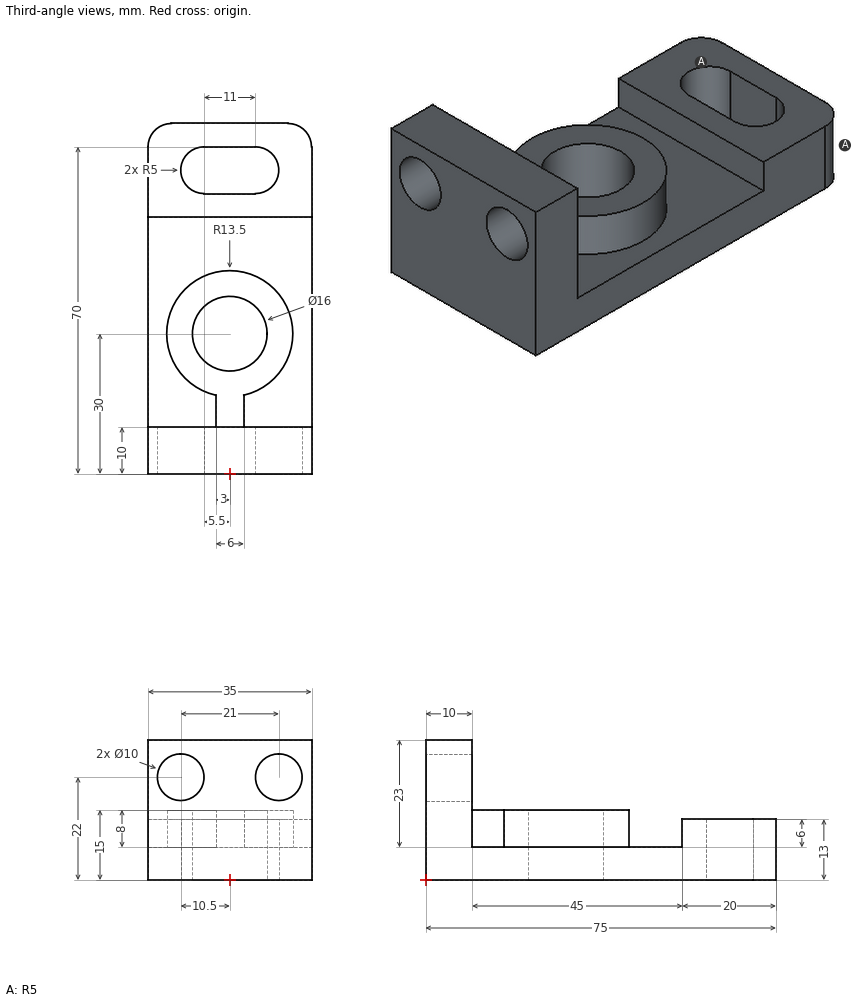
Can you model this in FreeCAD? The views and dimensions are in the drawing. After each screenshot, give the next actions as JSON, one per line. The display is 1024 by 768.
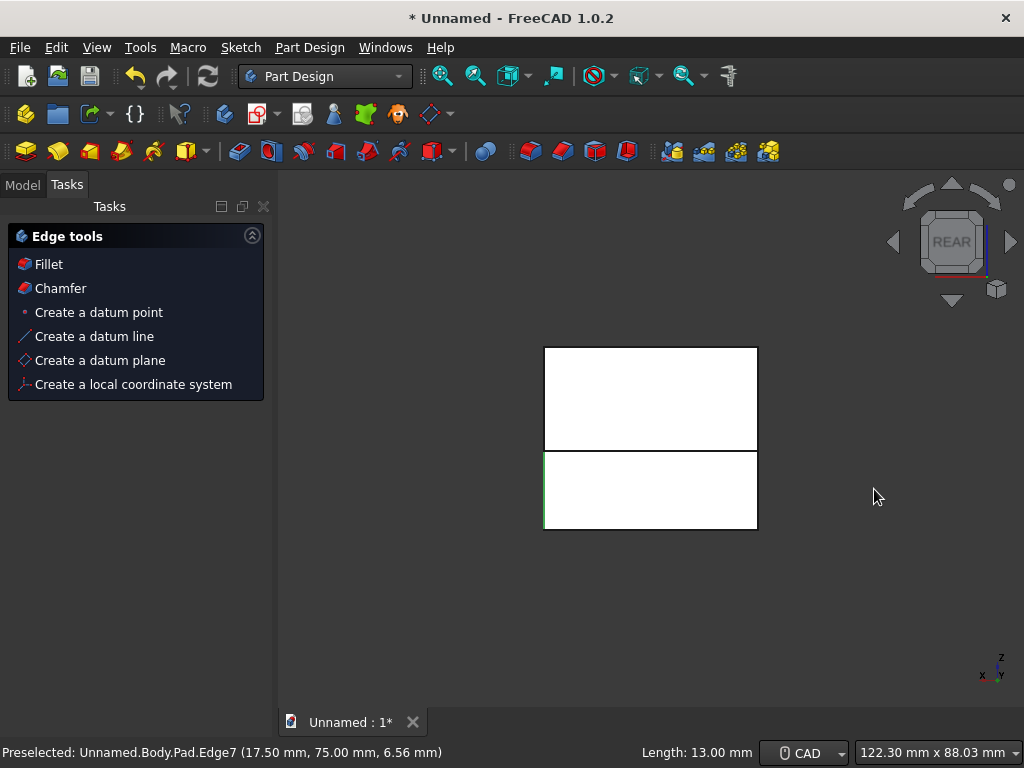
{"action": "key", "text": "v f"}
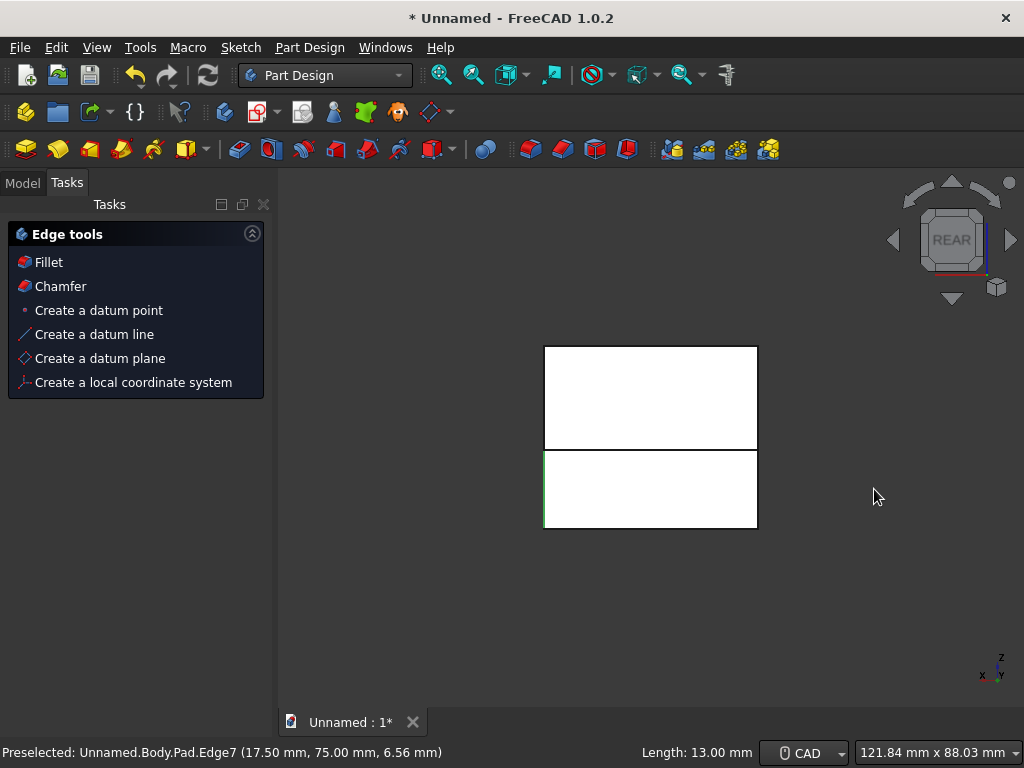
{"action": "left_click", "coordinate": [758, 489], "text": "ctrl"}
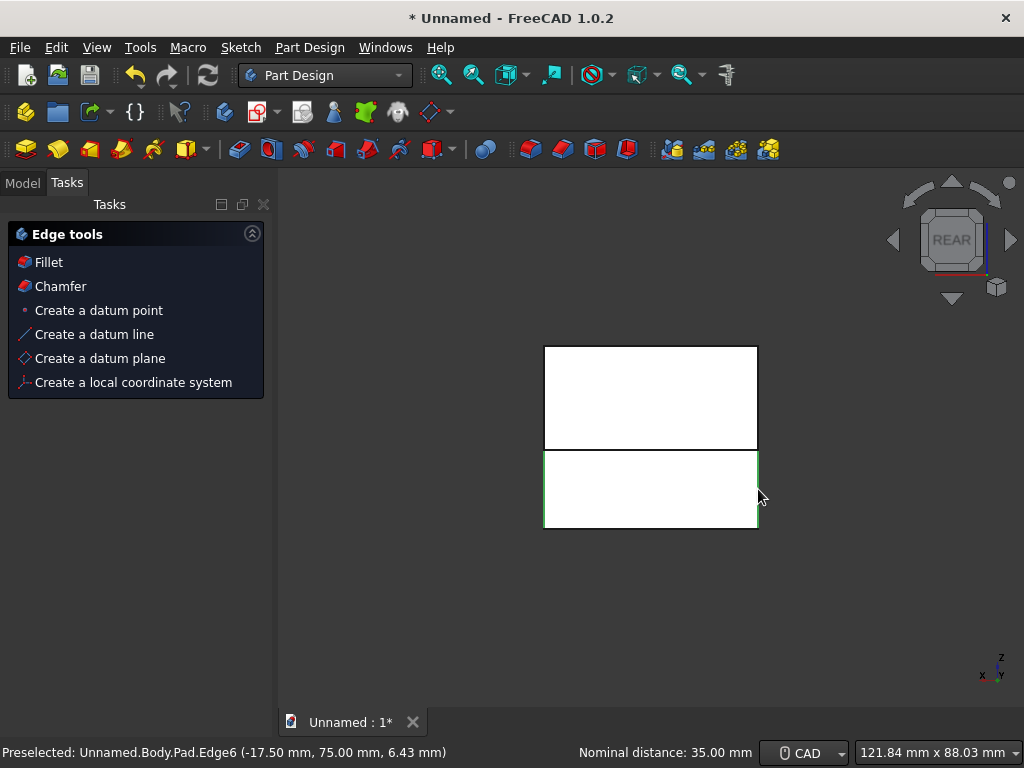
{"action": "left_click", "coordinate": [532, 150]}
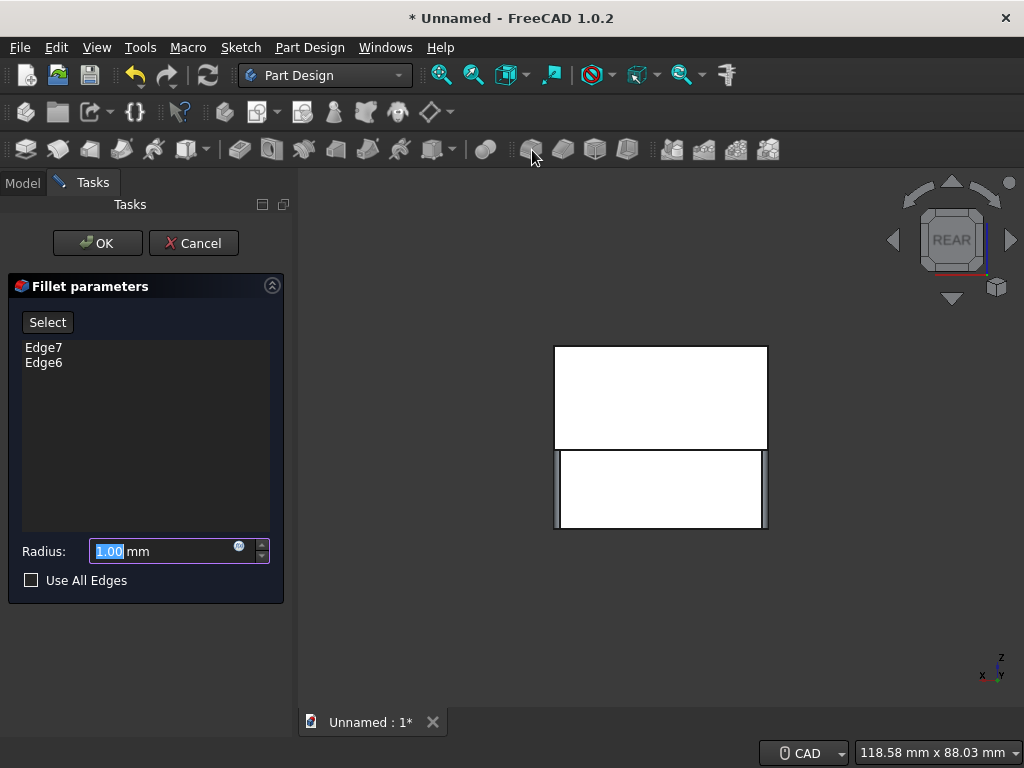
{"action": "type", "text": "5"}
{"action": "key", "text": "Tab"}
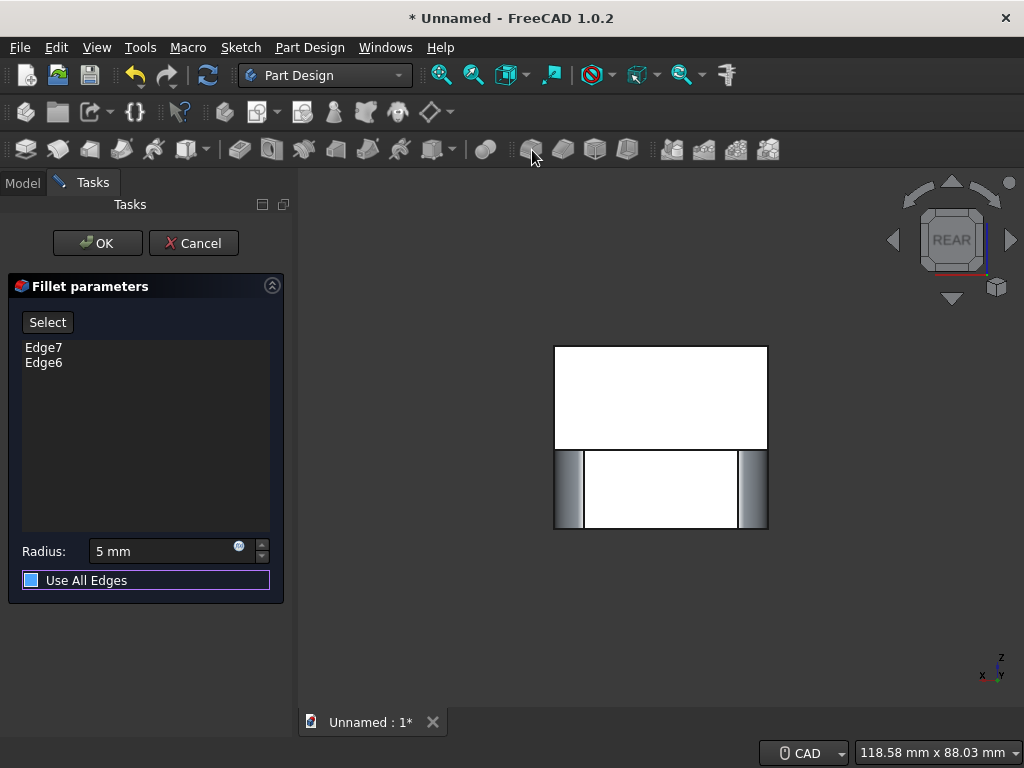
{"action": "left_click", "coordinate": [98, 243]}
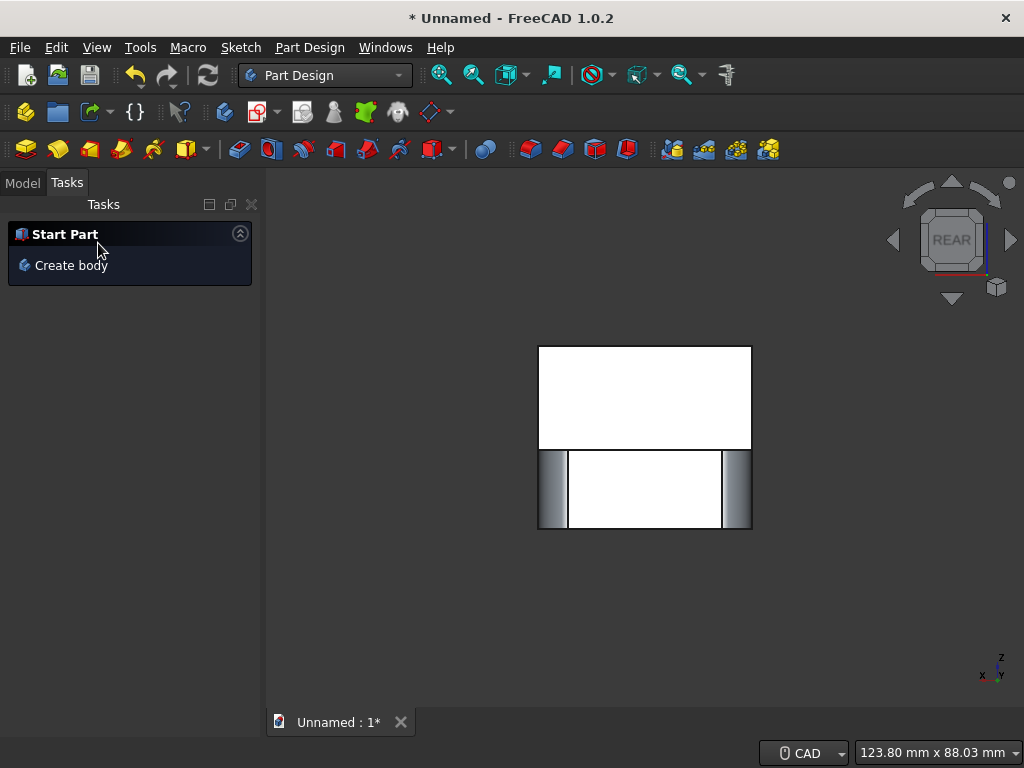
{"action": "key", "text": "v f"}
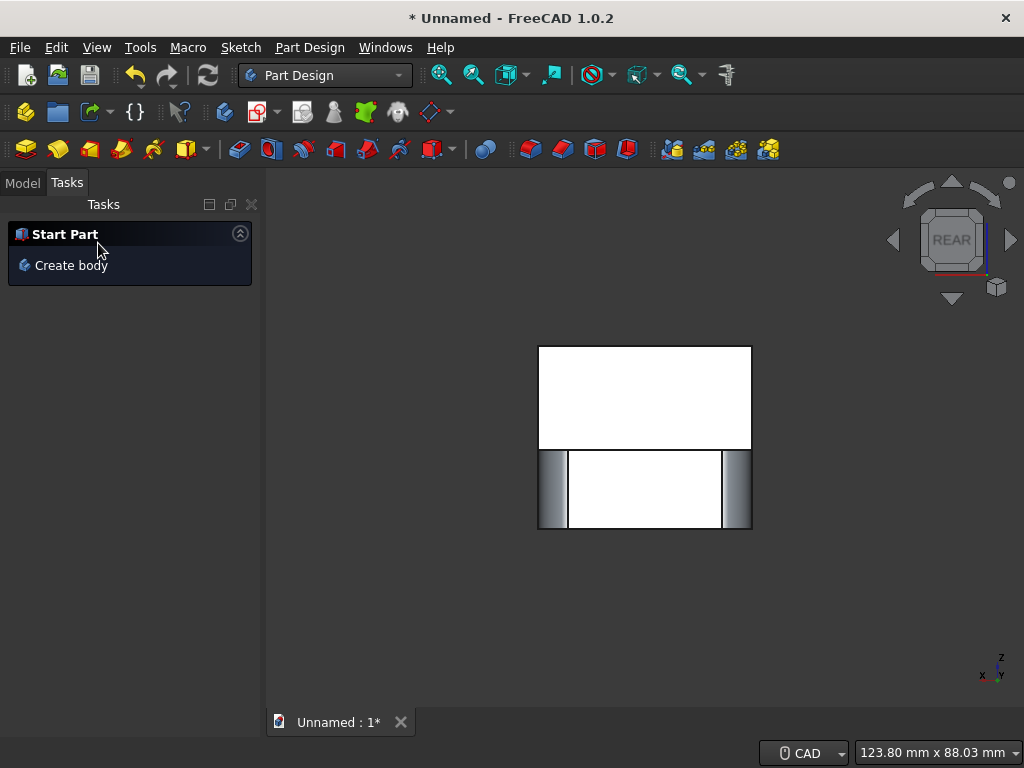
{"action": "key", "text": "0"}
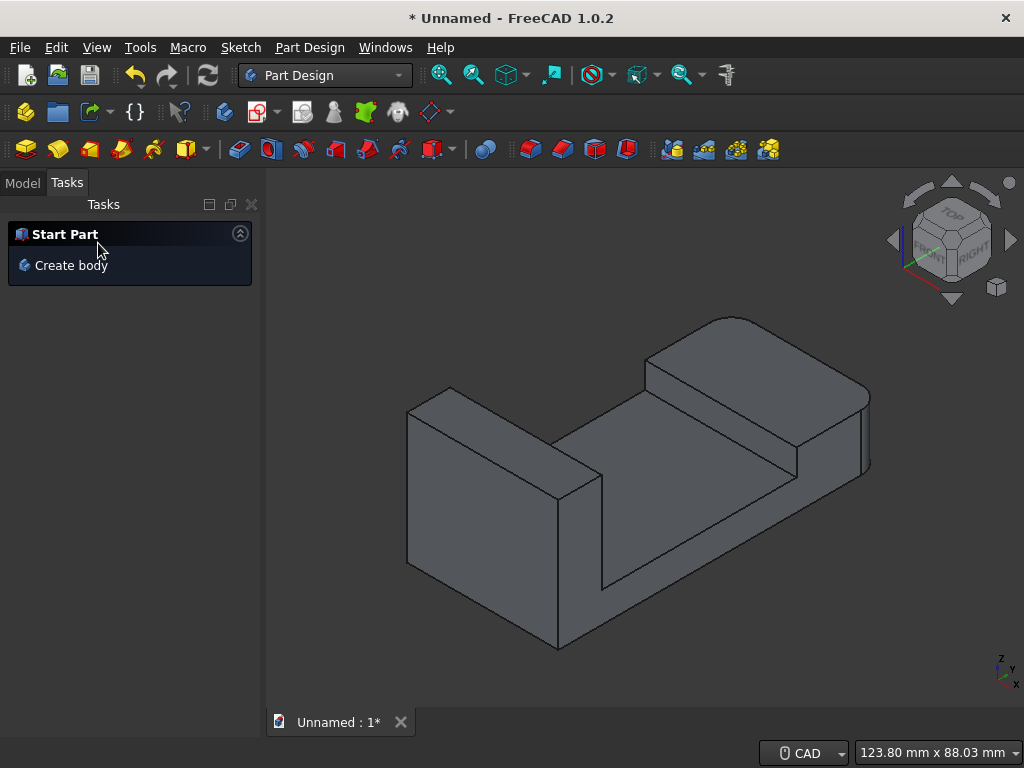
{"action": "left_click", "coordinate": [623, 489]}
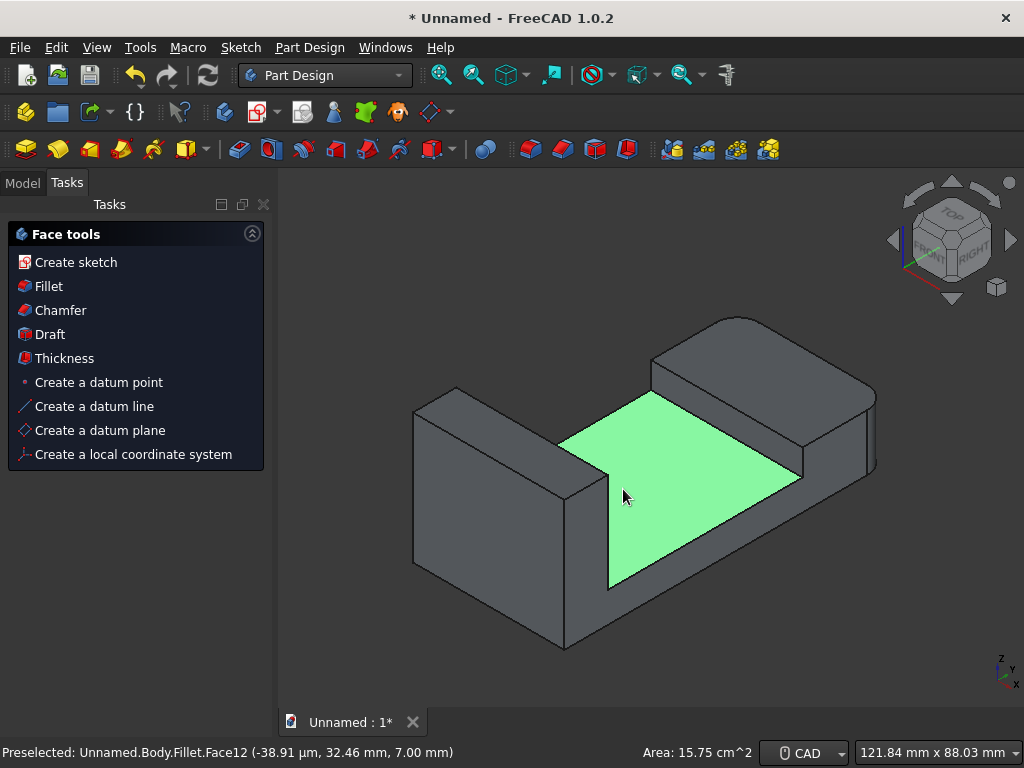
{"action": "left_click", "coordinate": [258, 112]}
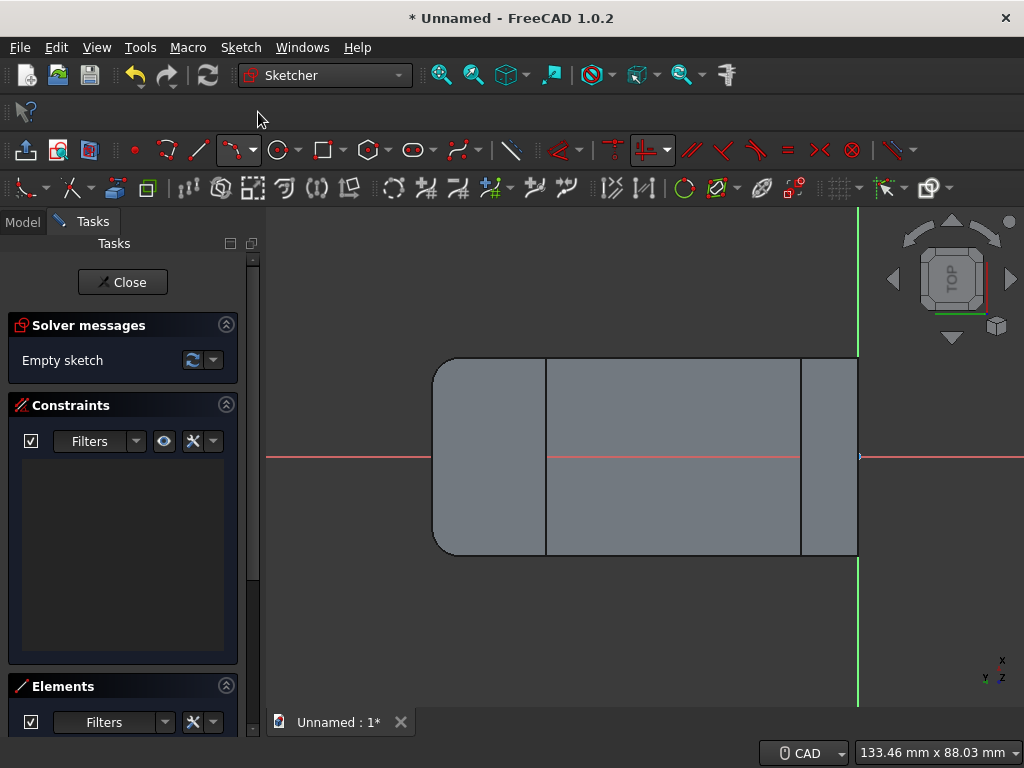
{"action": "left_click", "coordinate": [90, 150]}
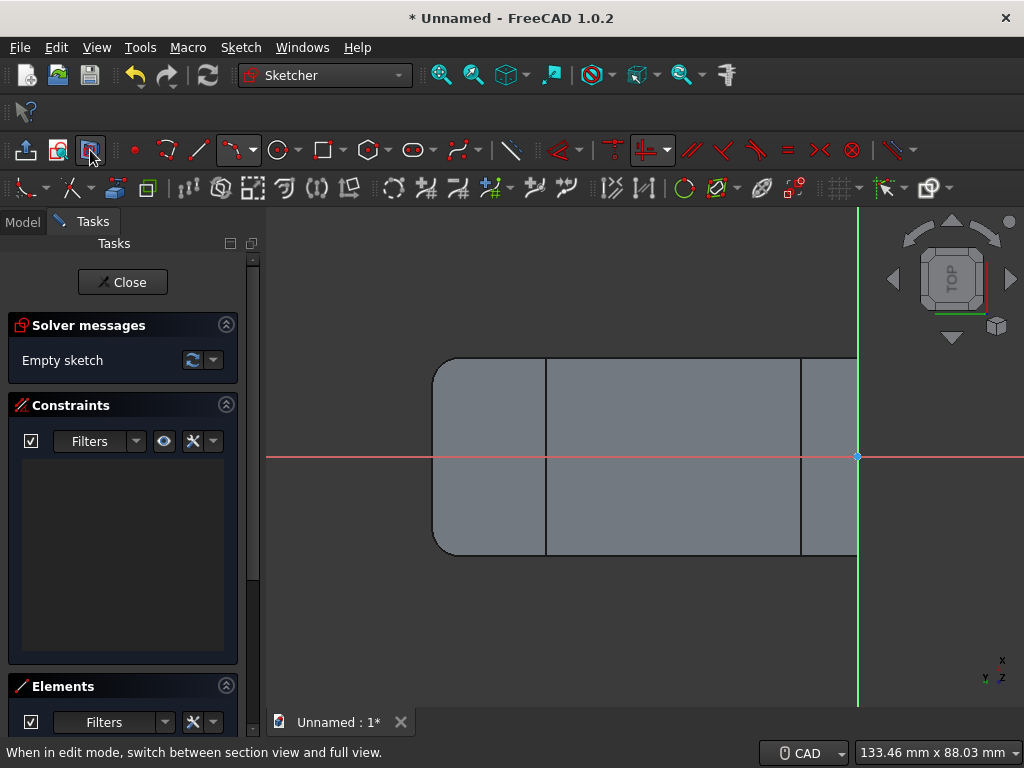
{"action": "scroll", "coordinate": [294, 457], "scroll_direction": "down", "scroll_amount": 1}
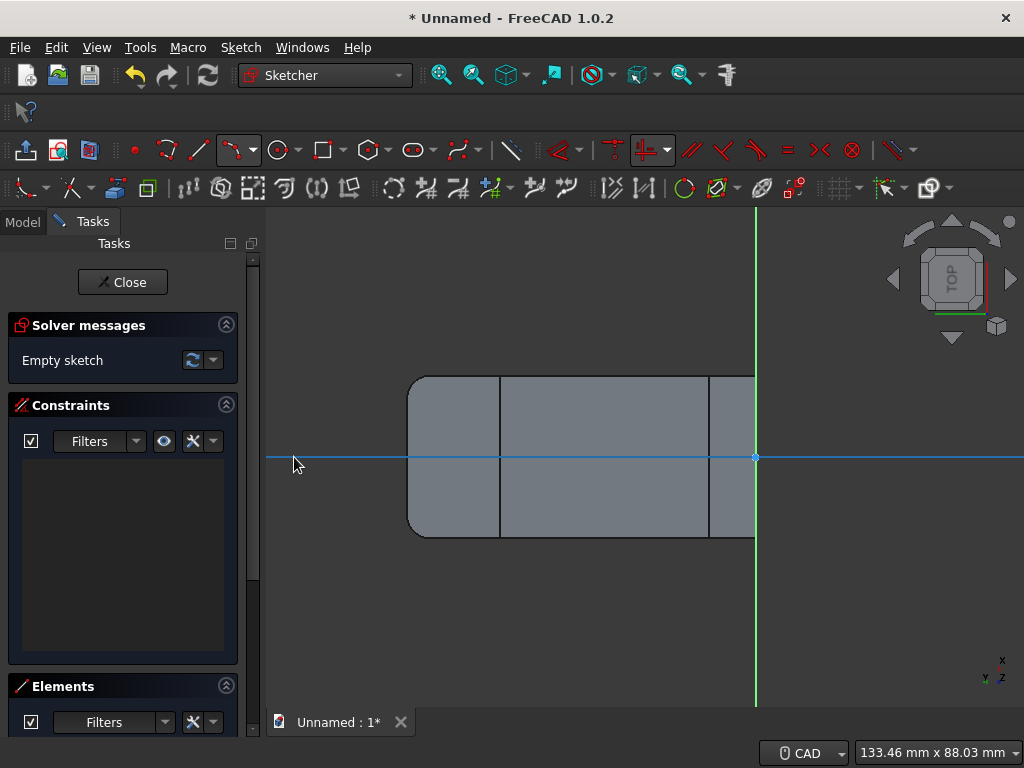
{"action": "scroll", "coordinate": [750, 457], "scroll_direction": "up", "scroll_amount": 3}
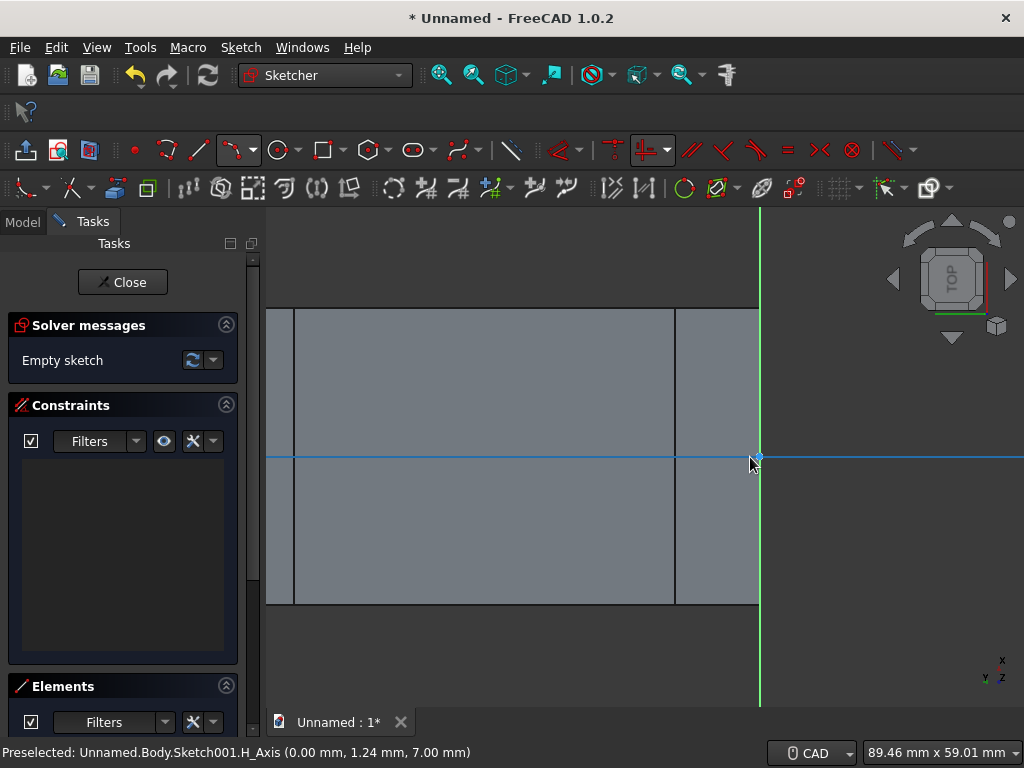
{"action": "key", "text": "g m"}